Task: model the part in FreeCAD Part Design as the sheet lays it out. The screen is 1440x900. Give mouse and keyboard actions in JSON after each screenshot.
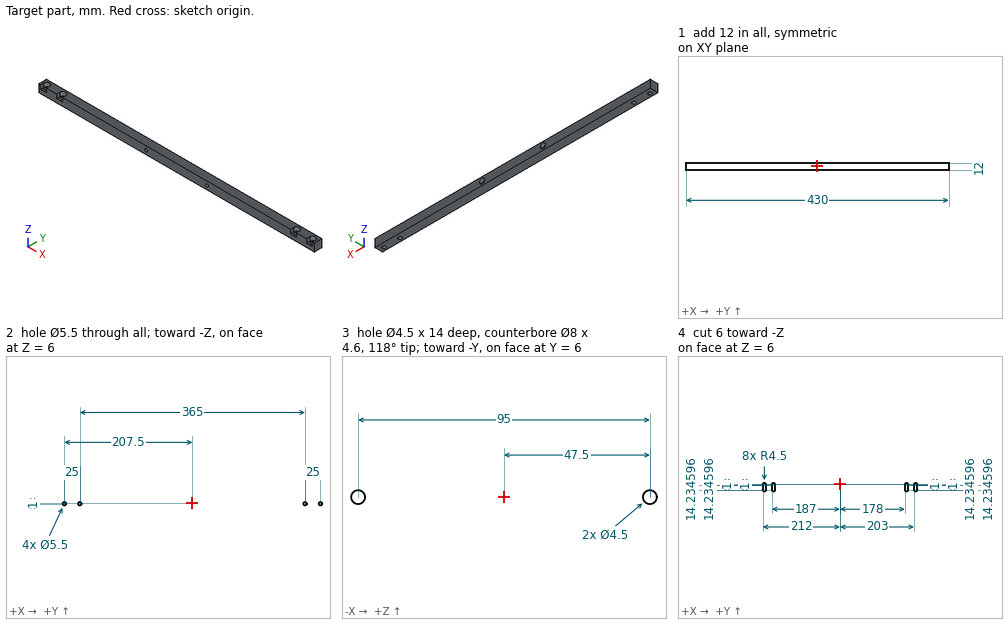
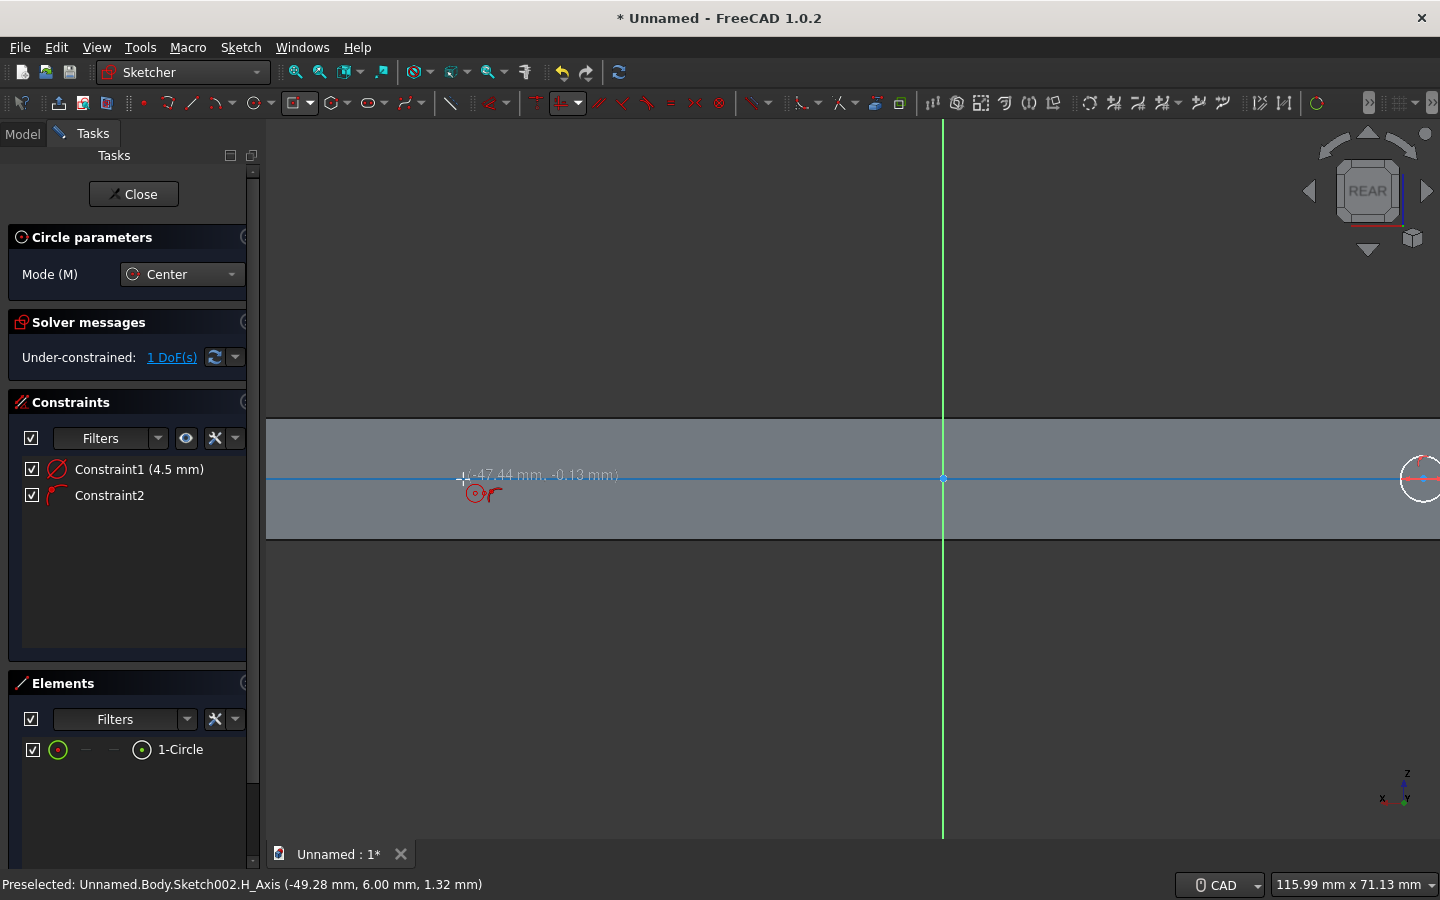
{"action": "left_click", "coordinate": [462, 479]}
{"action": "mouse_move", "coordinate": [478, 463]}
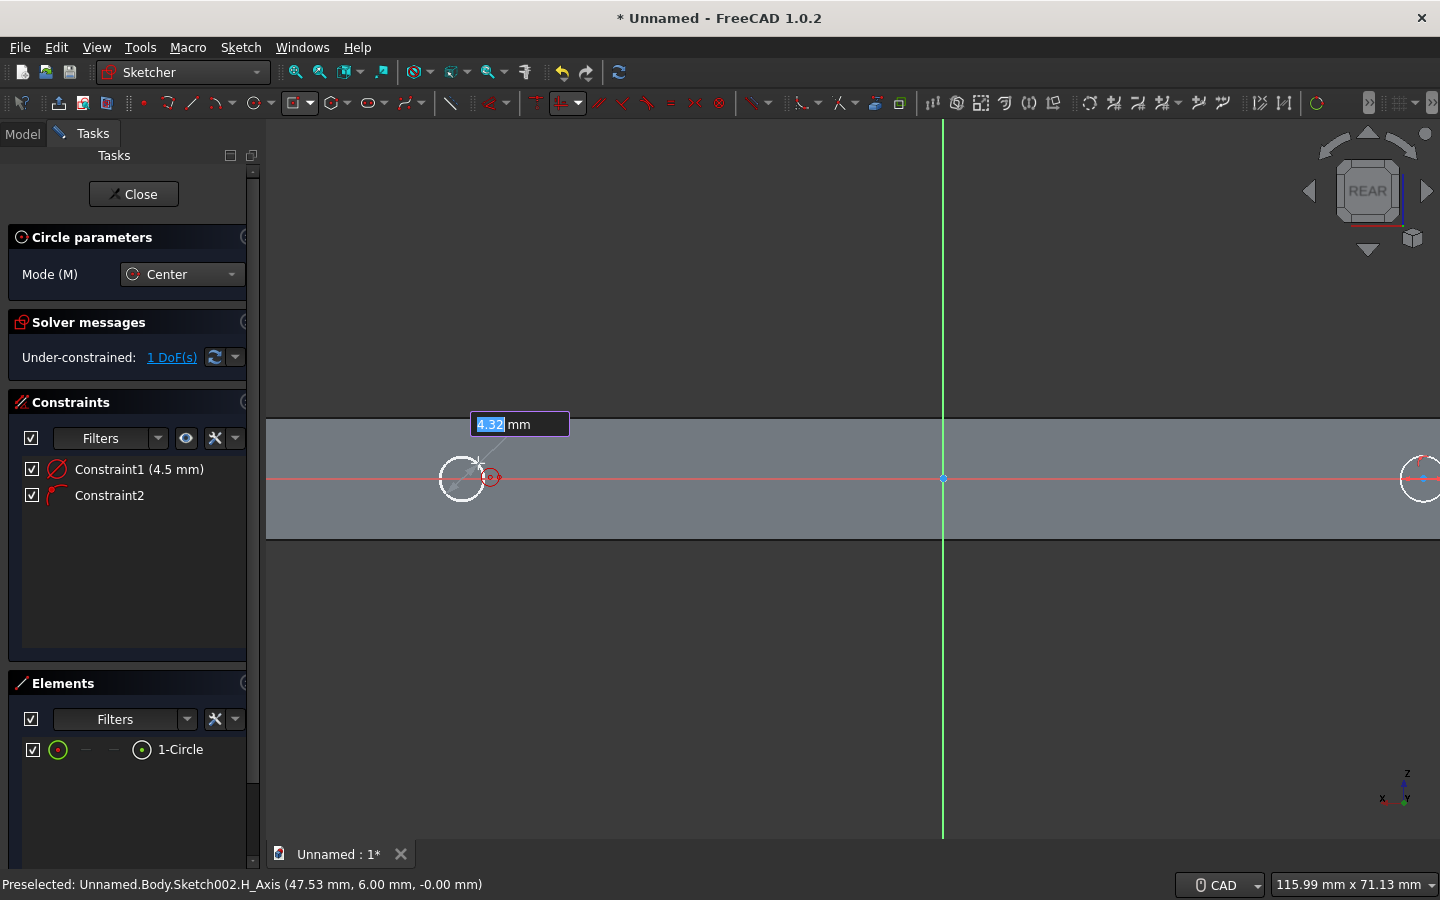
{"action": "type", "text": "4.5"}
{"action": "key", "text": "Return"}
{"action": "key", "text": "Escape"}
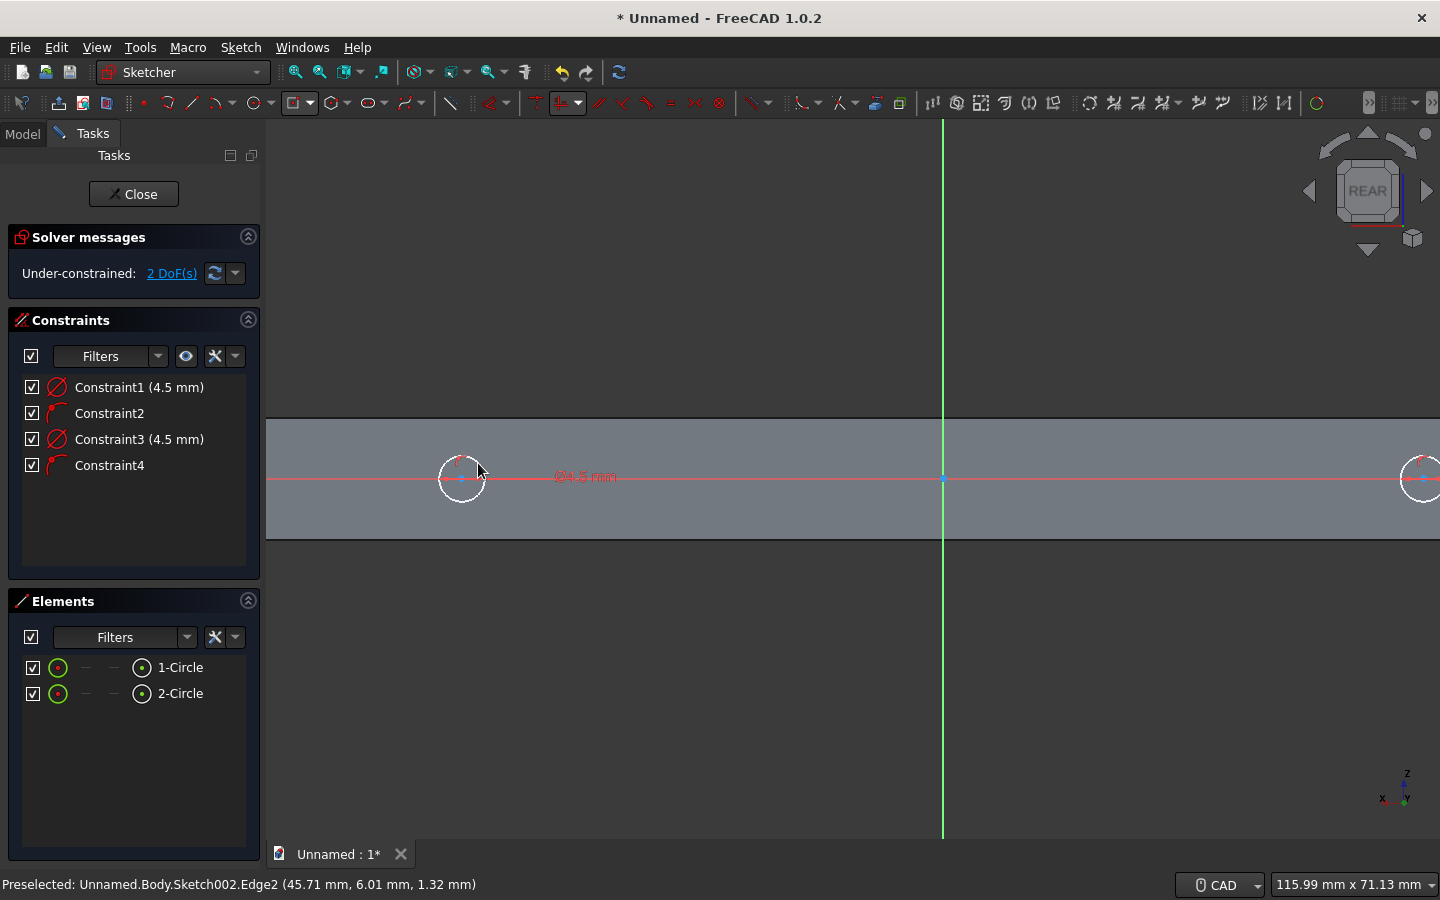
{"action": "left_click", "coordinate": [490, 104]}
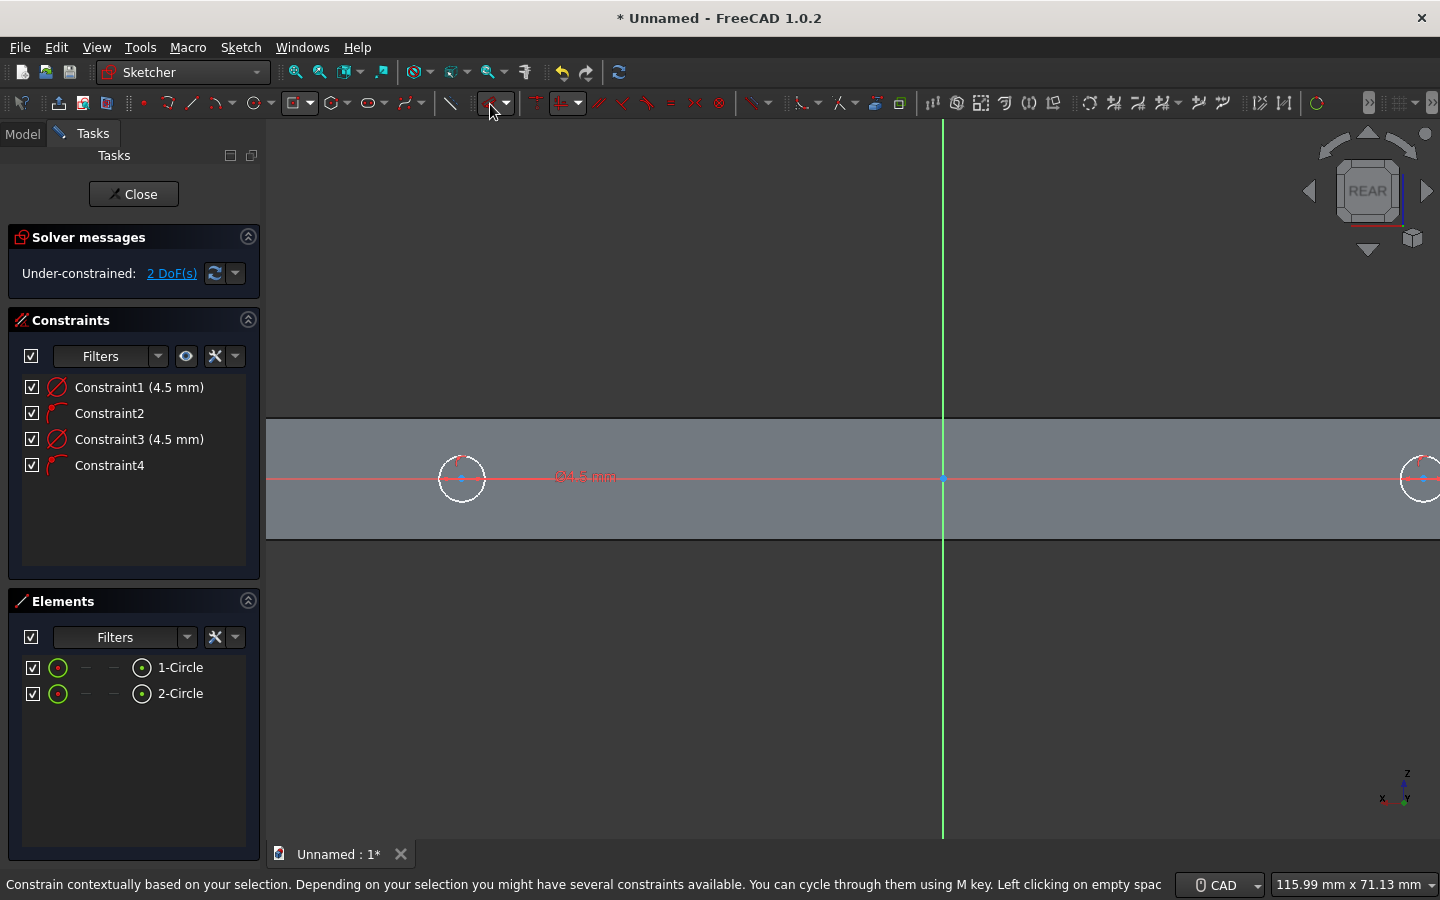
{"action": "scroll", "coordinate": [462, 479], "scroll_direction": "down", "scroll_amount": 2}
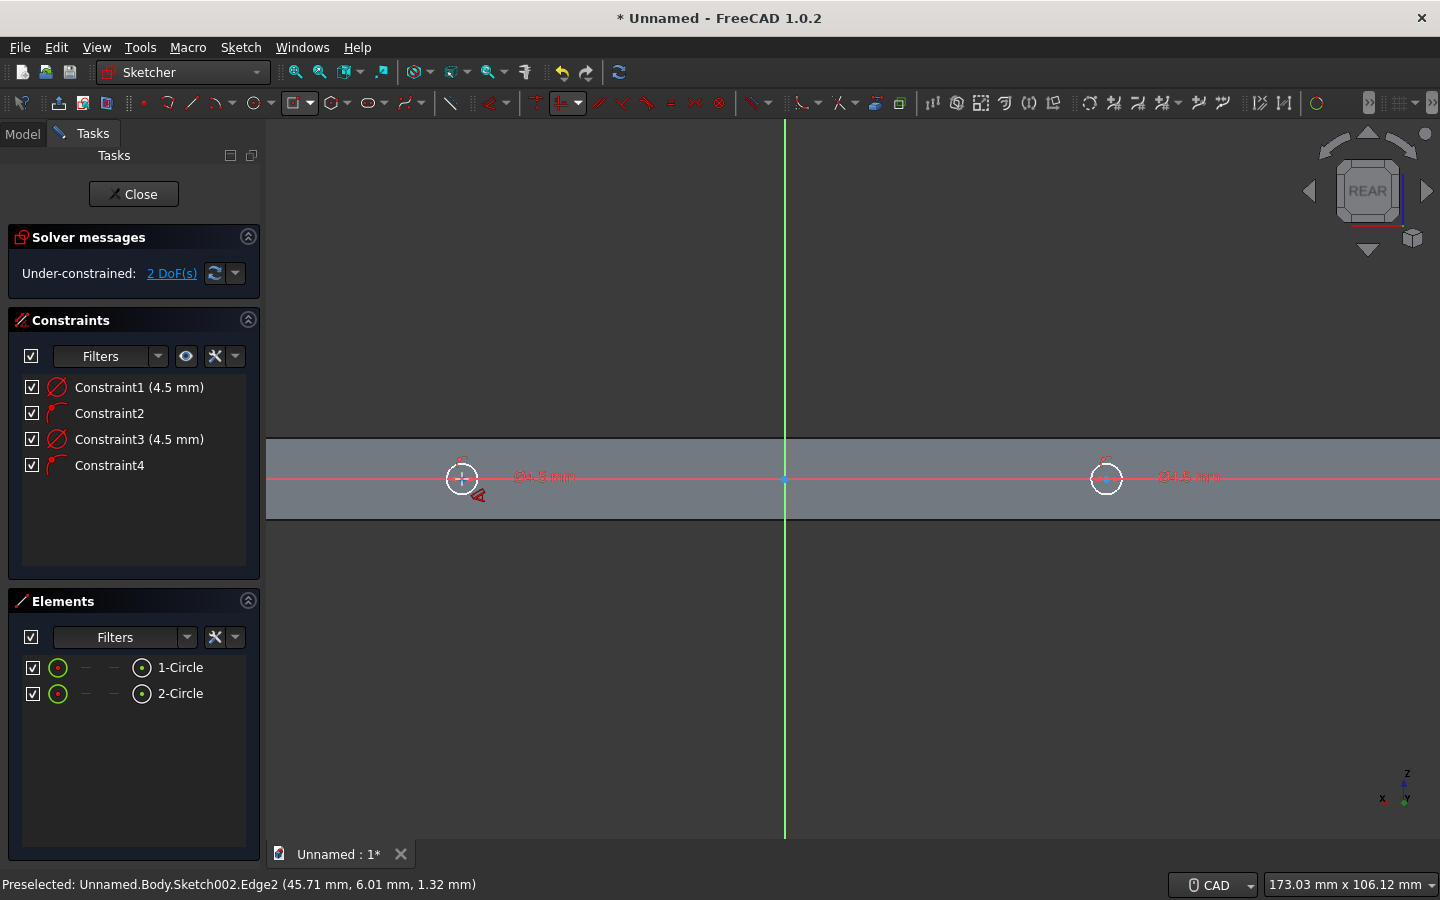
{"action": "left_click", "coordinate": [1107, 479]}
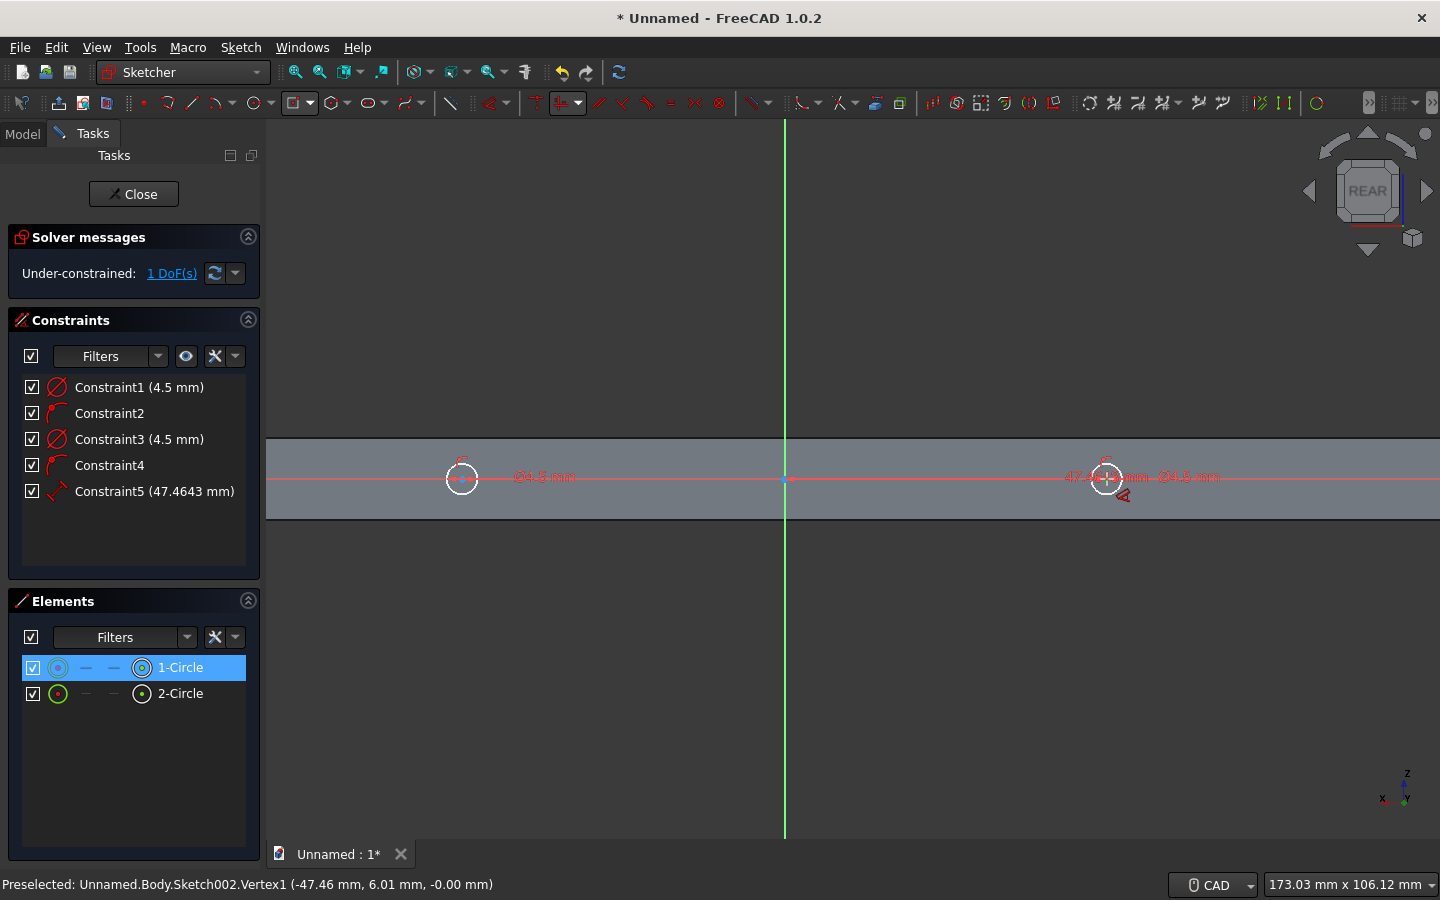
{"action": "left_click", "coordinate": [462, 479]}
{"action": "left_click", "coordinate": [636, 513]}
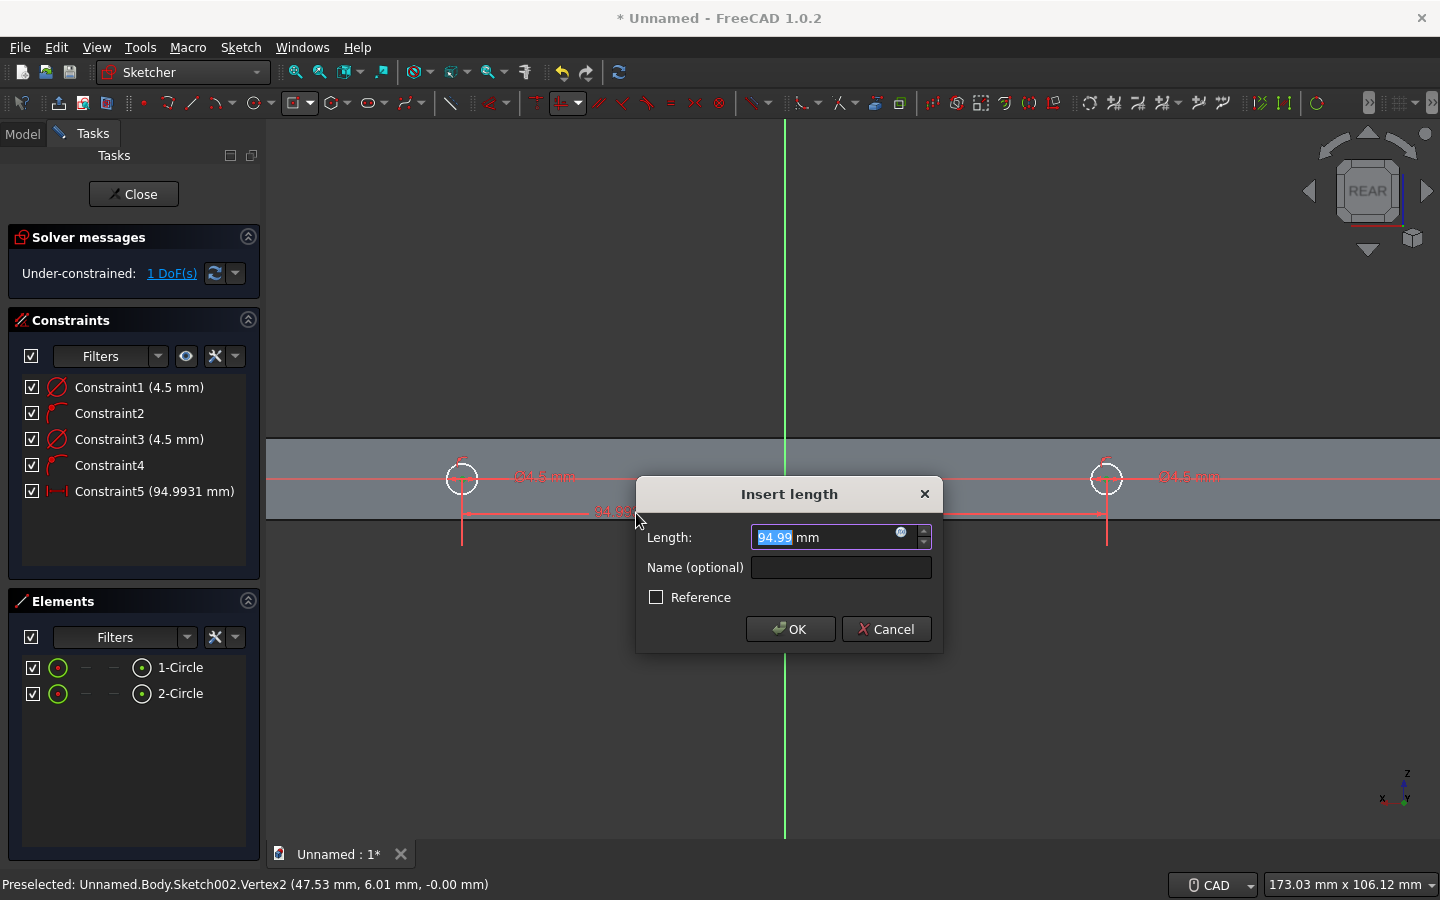
{"action": "type", "text": "95"}
{"action": "key", "text": "Return"}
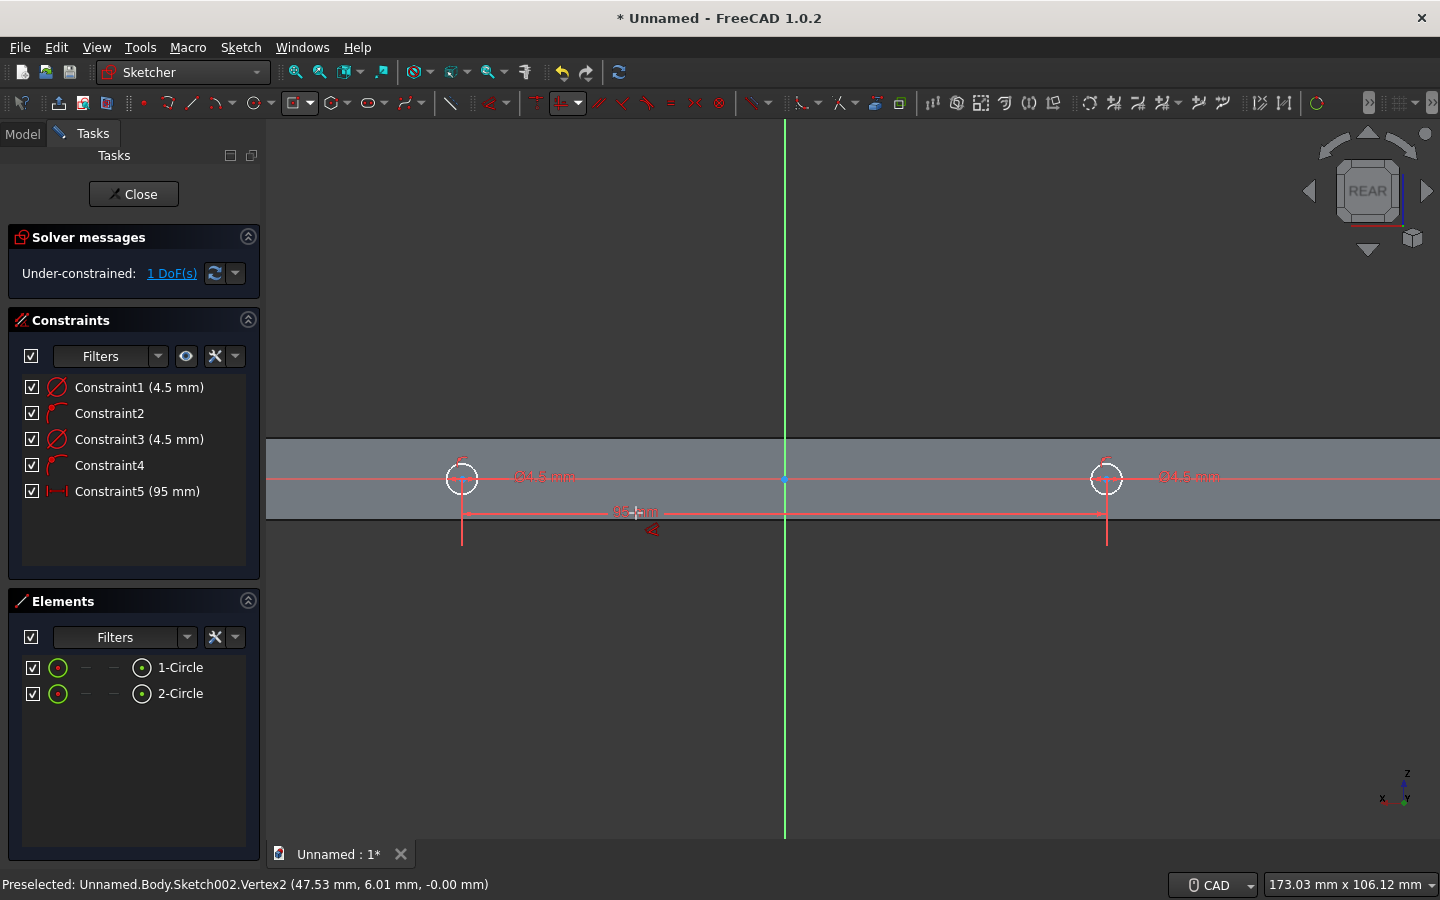
{"action": "left_click", "coordinate": [1107, 479]}
{"action": "left_click", "coordinate": [946, 513]}